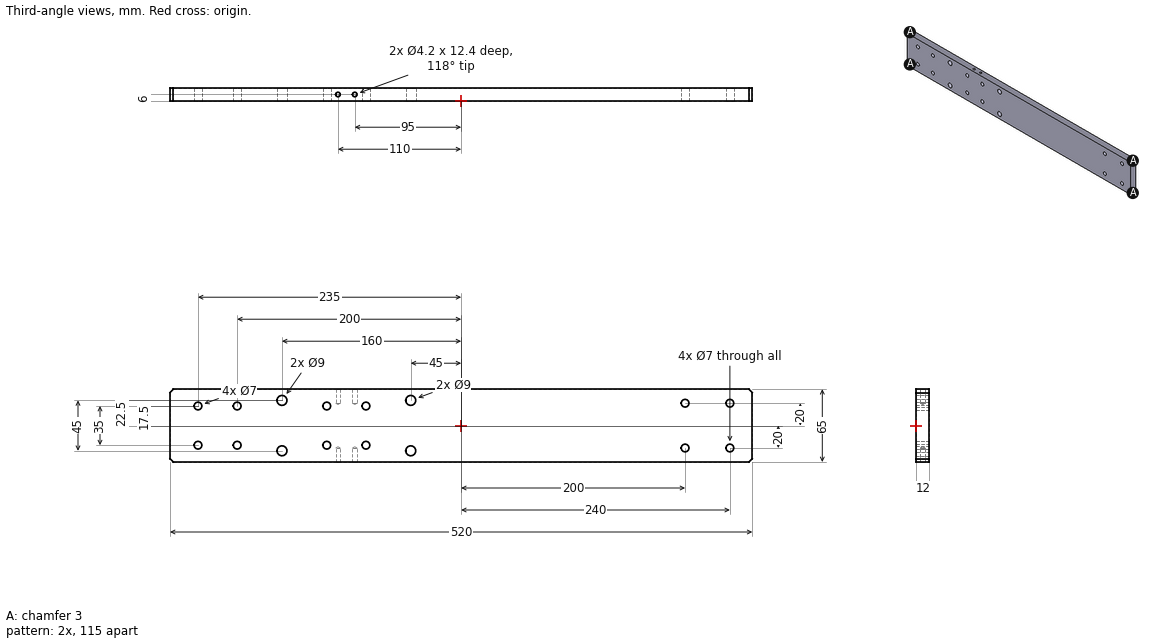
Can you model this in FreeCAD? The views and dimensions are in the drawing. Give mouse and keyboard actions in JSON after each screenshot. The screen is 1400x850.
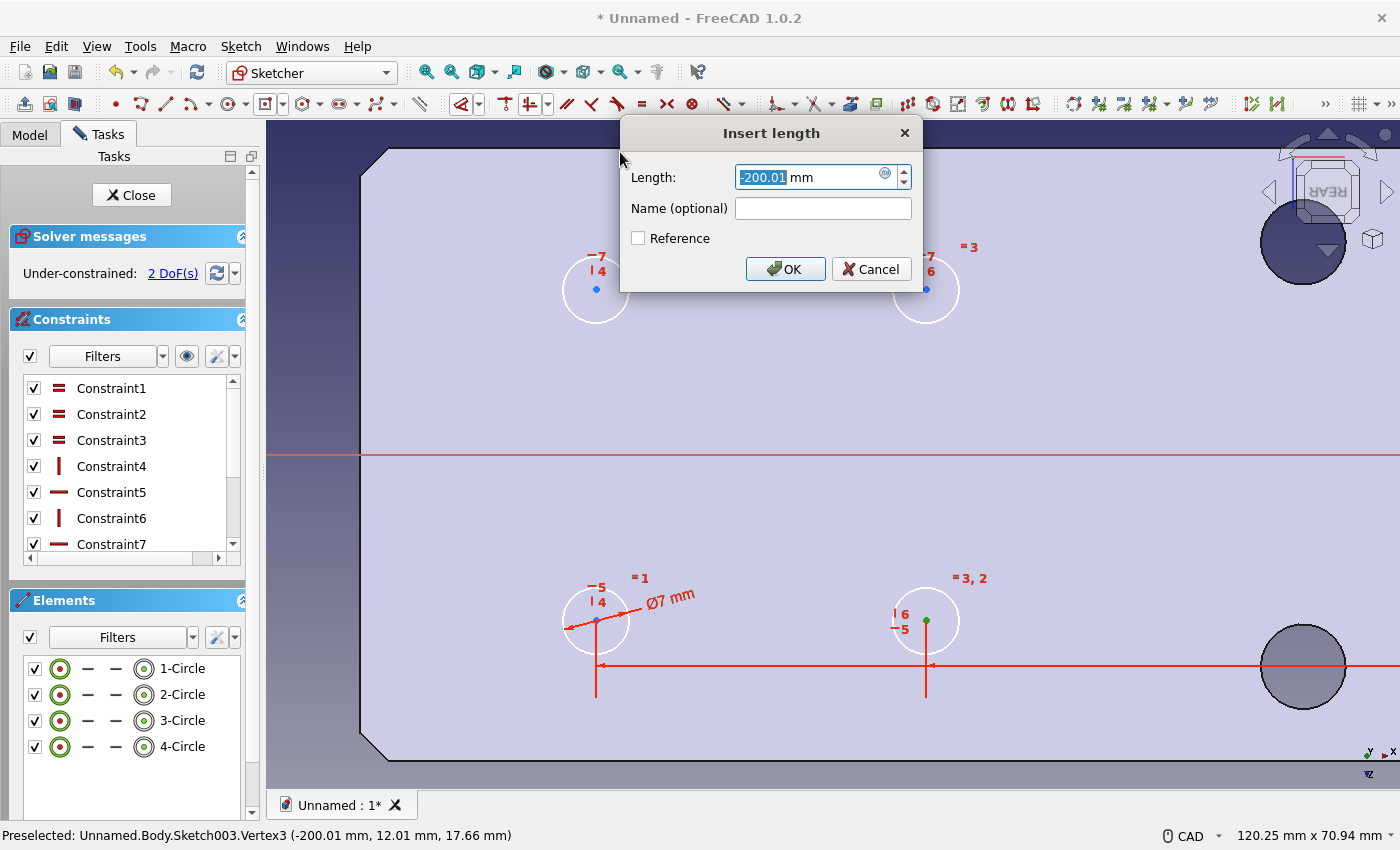
{"action": "type", "text": "-200"}
{"action": "key", "text": "Return"}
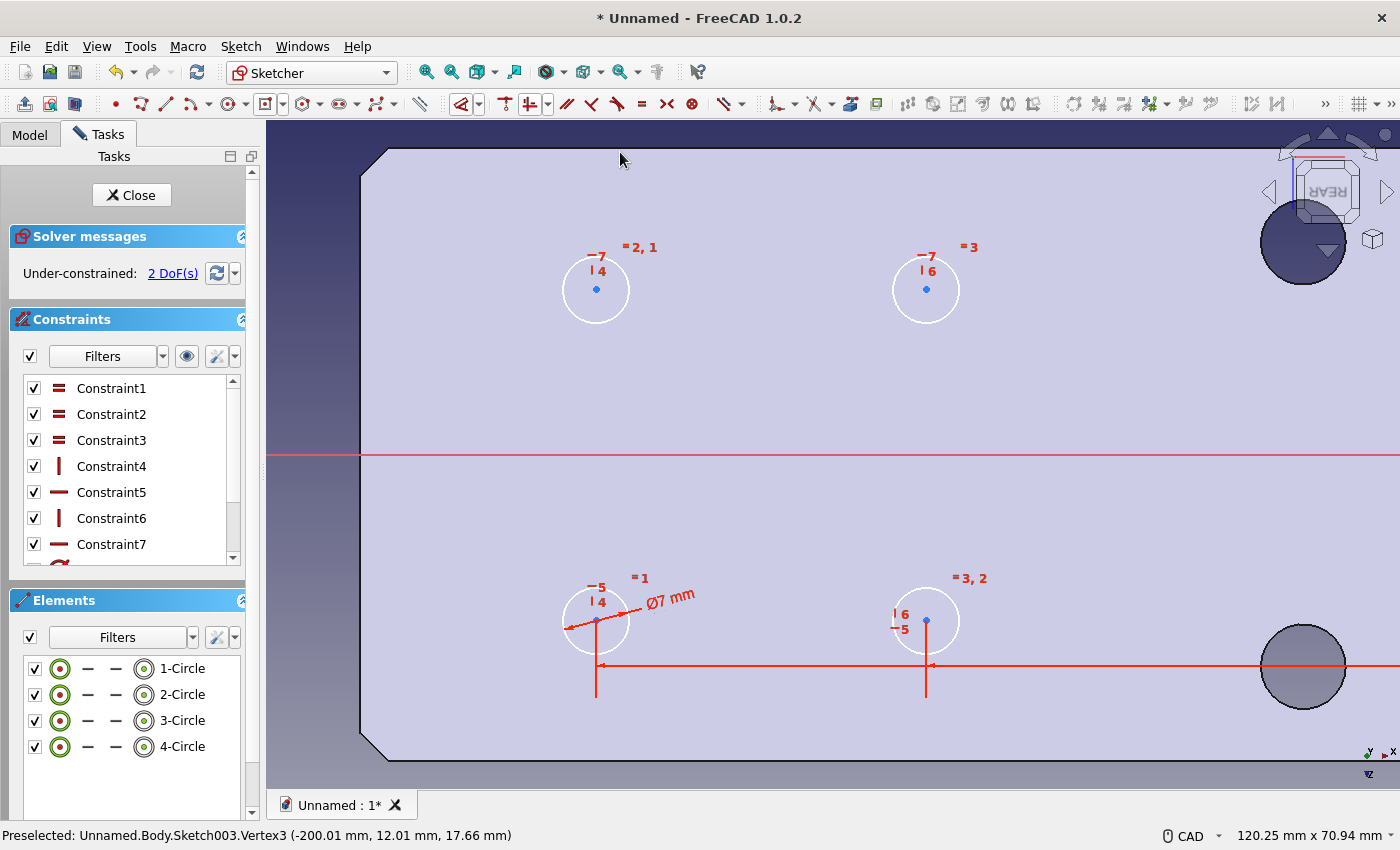
{"action": "left_click", "coordinate": [596, 621]}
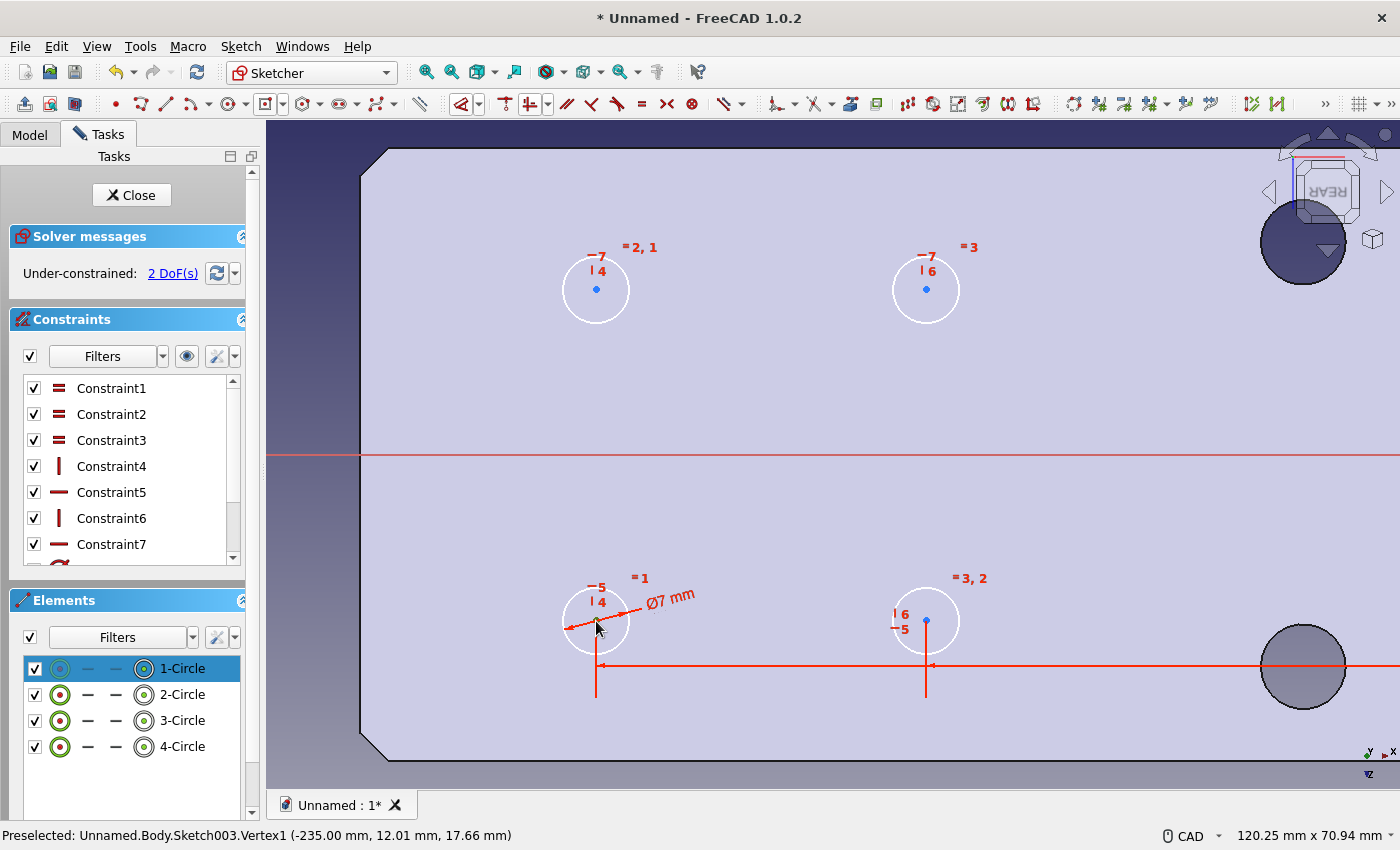
{"action": "left_click", "coordinate": [596, 290]}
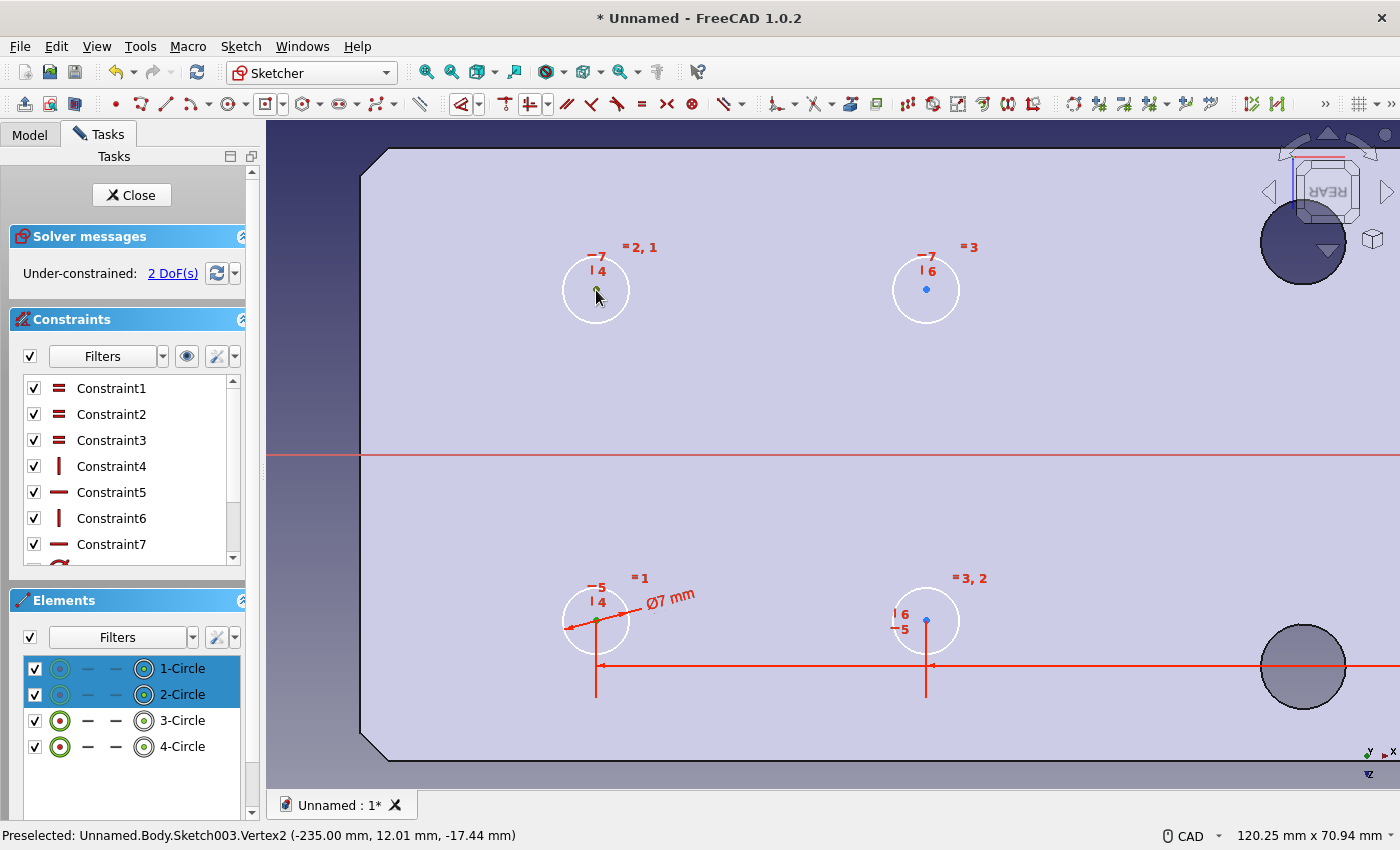
{"action": "left_click", "coordinate": [478, 104]}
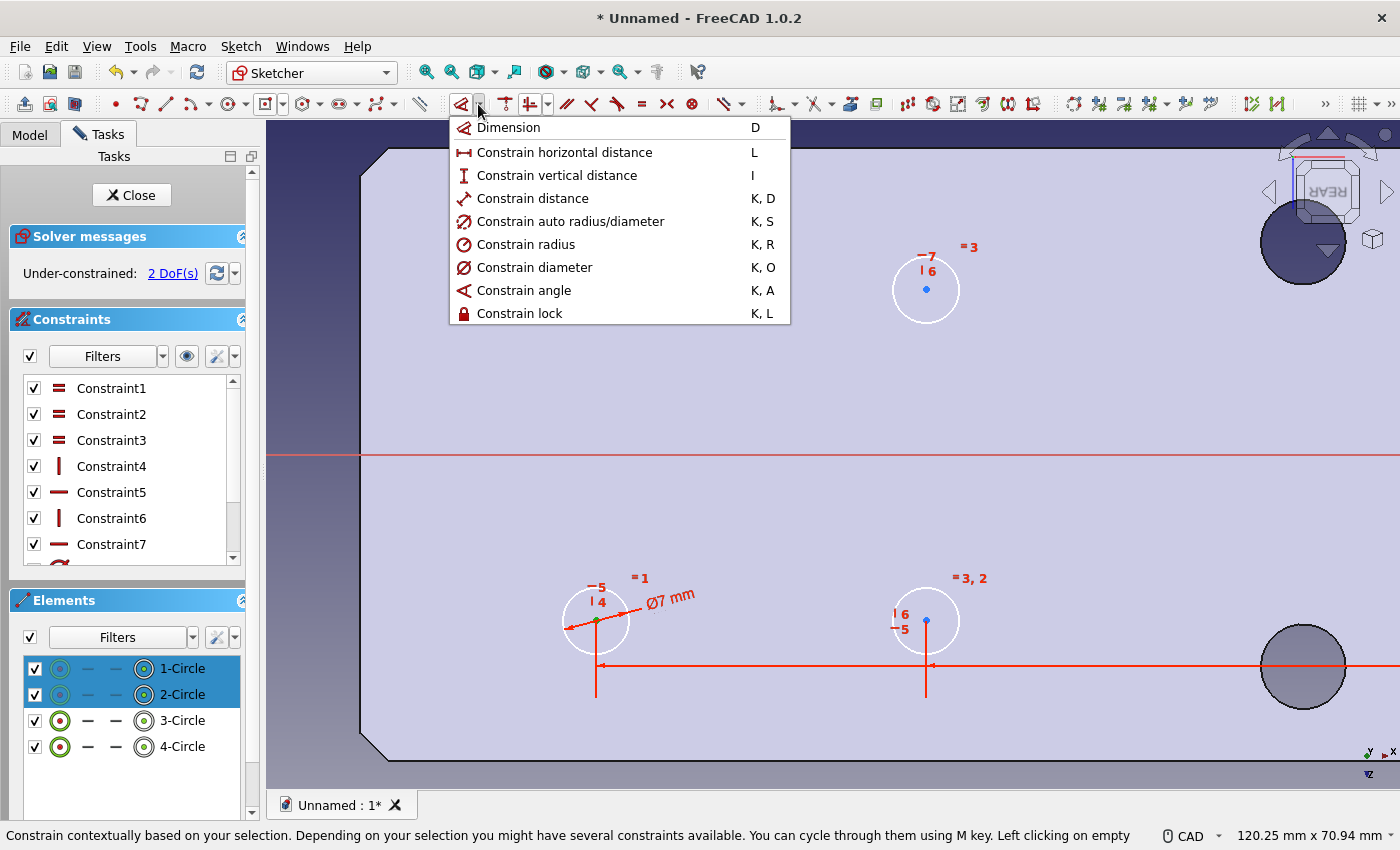
{"action": "left_click", "coordinate": [620, 176]}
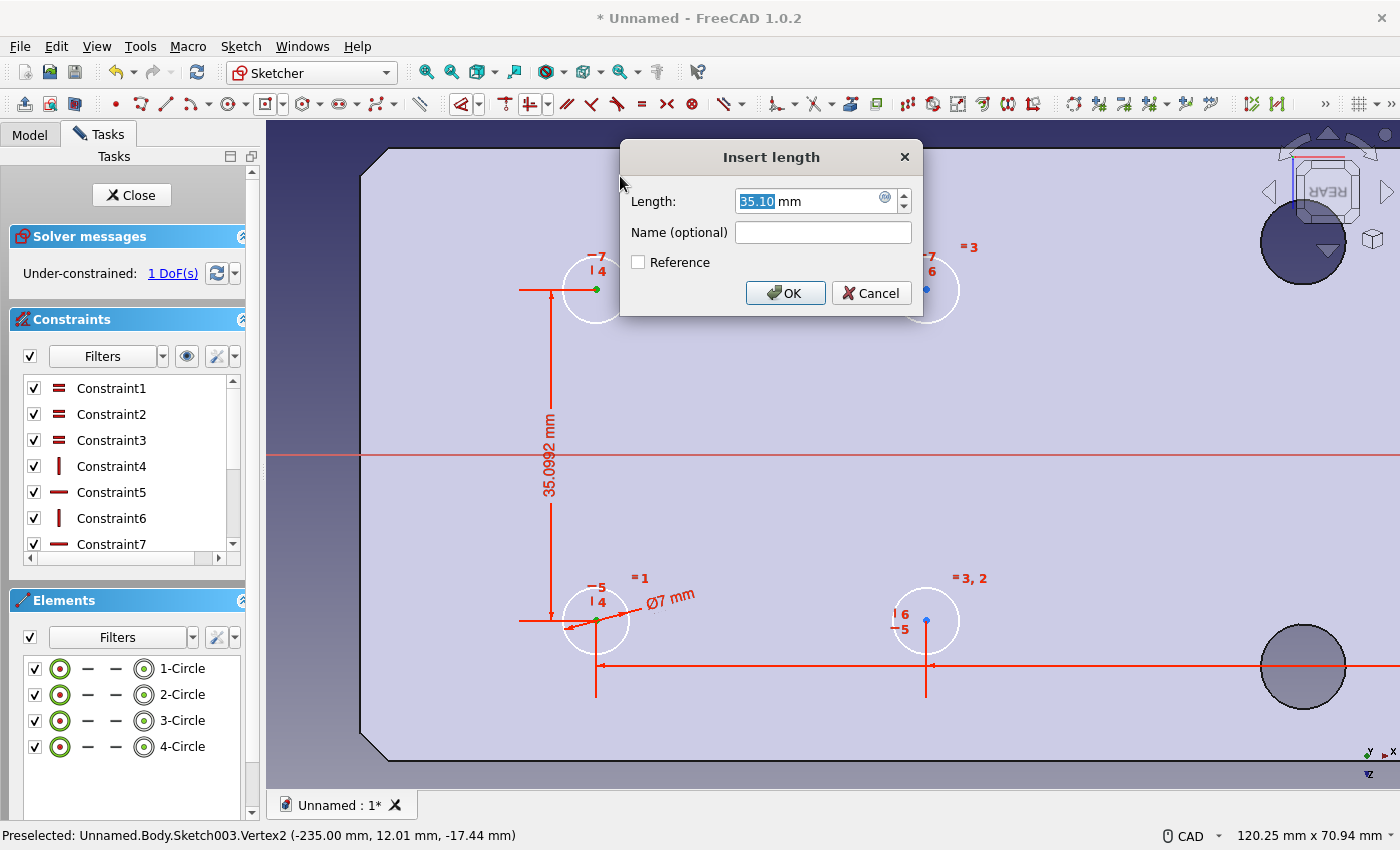
{"action": "type", "text": "35"}
{"action": "key", "text": "Return"}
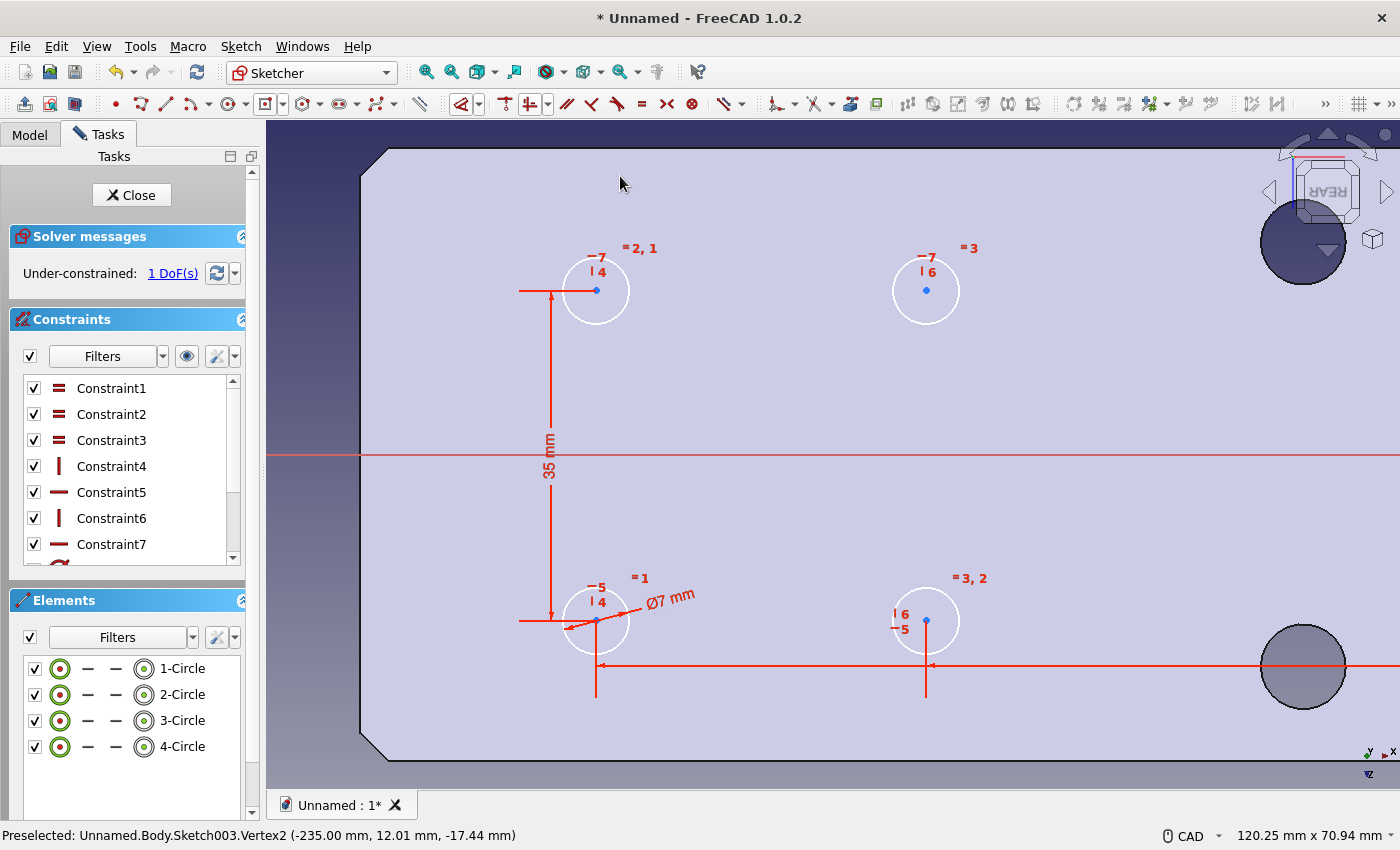
{"action": "left_click", "coordinate": [596, 621]}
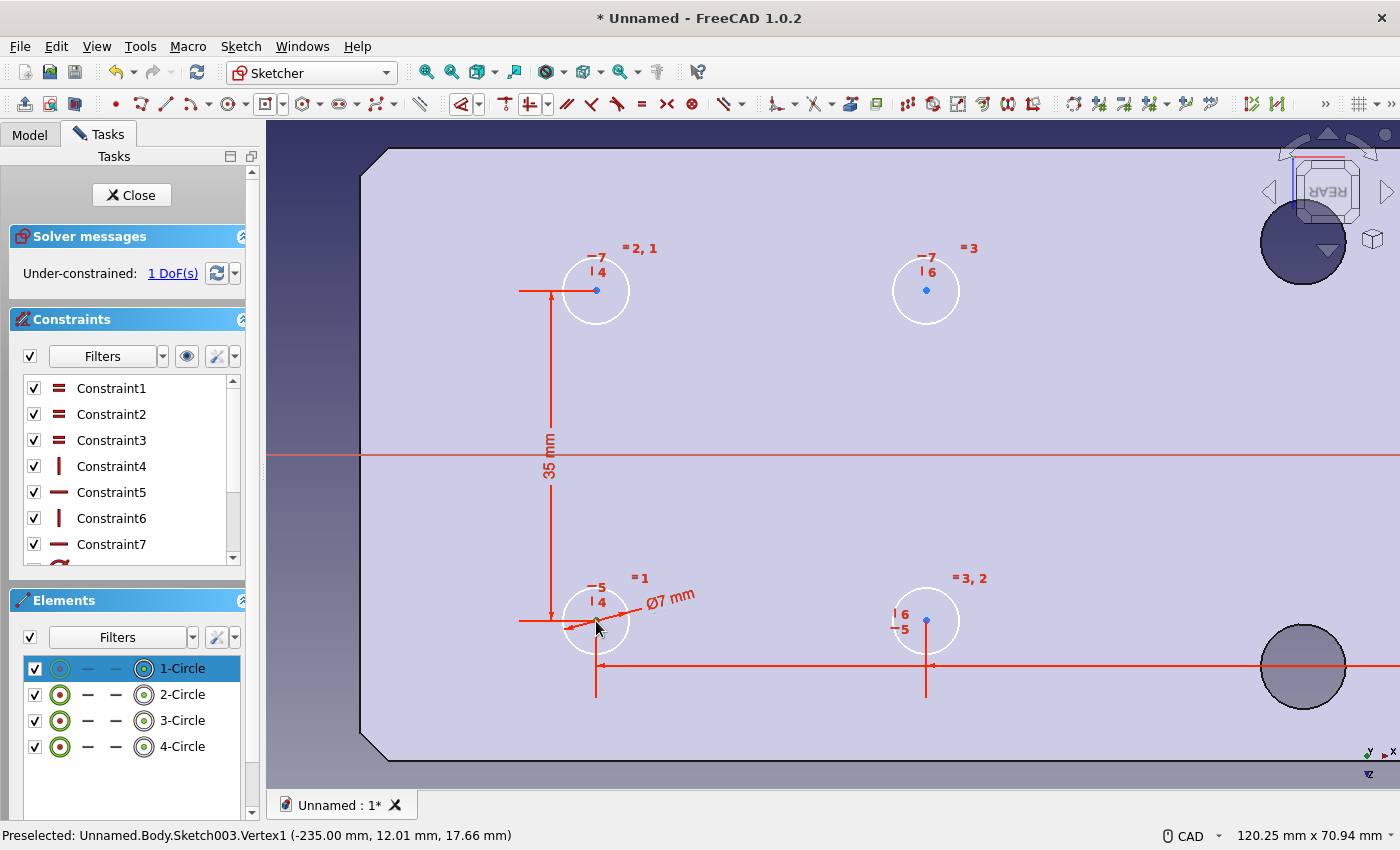
{"action": "left_click", "coordinate": [478, 104]}